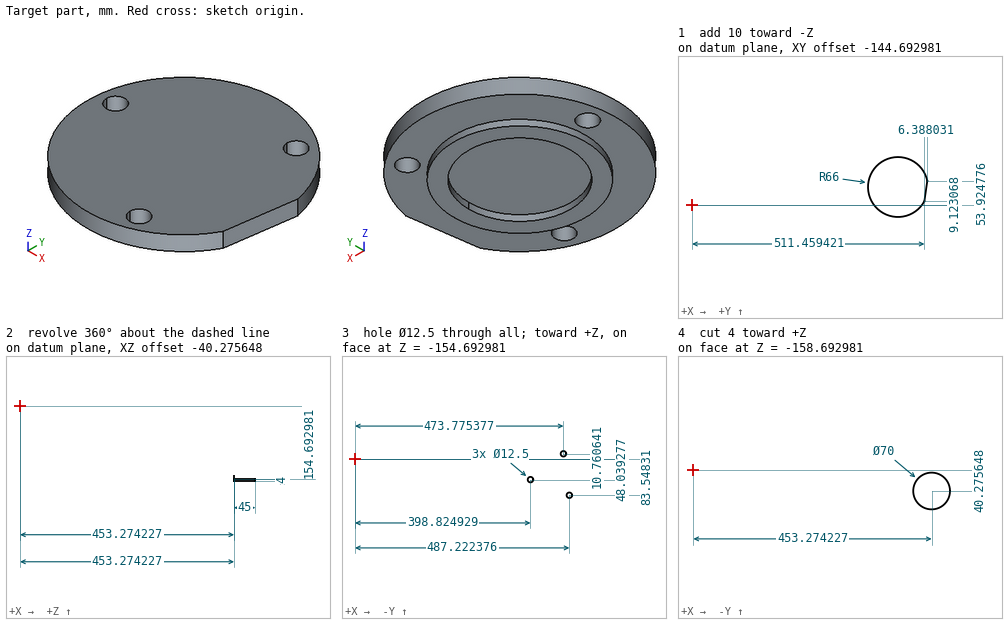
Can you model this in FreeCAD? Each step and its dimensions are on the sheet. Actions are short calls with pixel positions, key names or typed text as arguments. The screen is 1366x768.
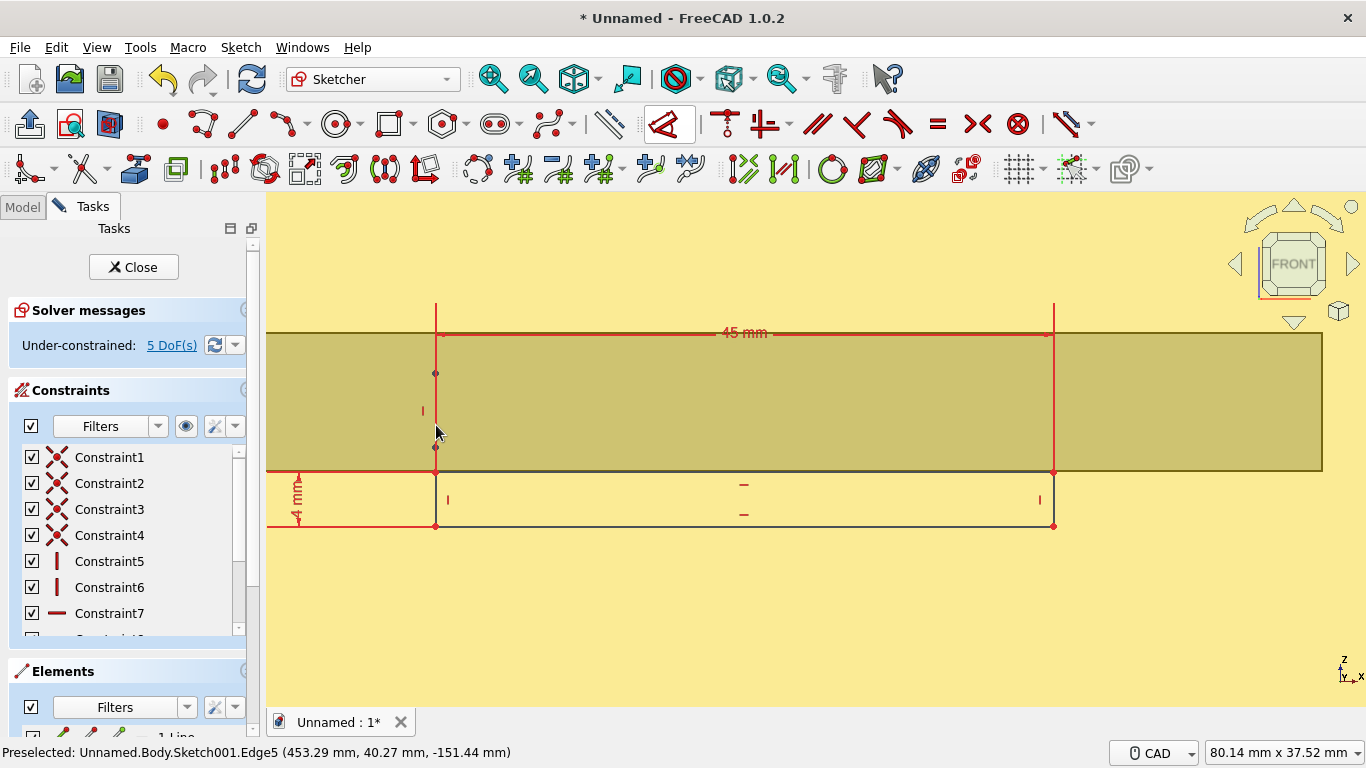
key(g)
key(n)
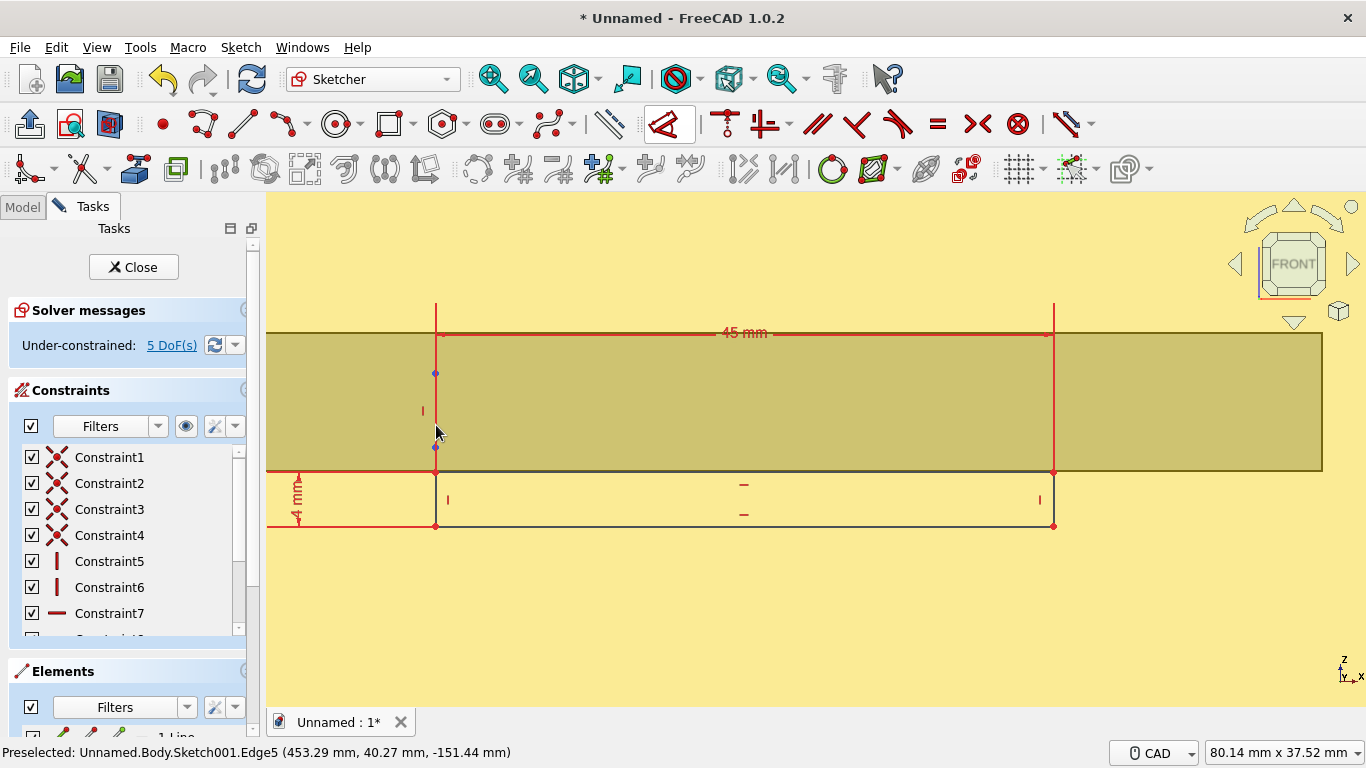
click(436, 472)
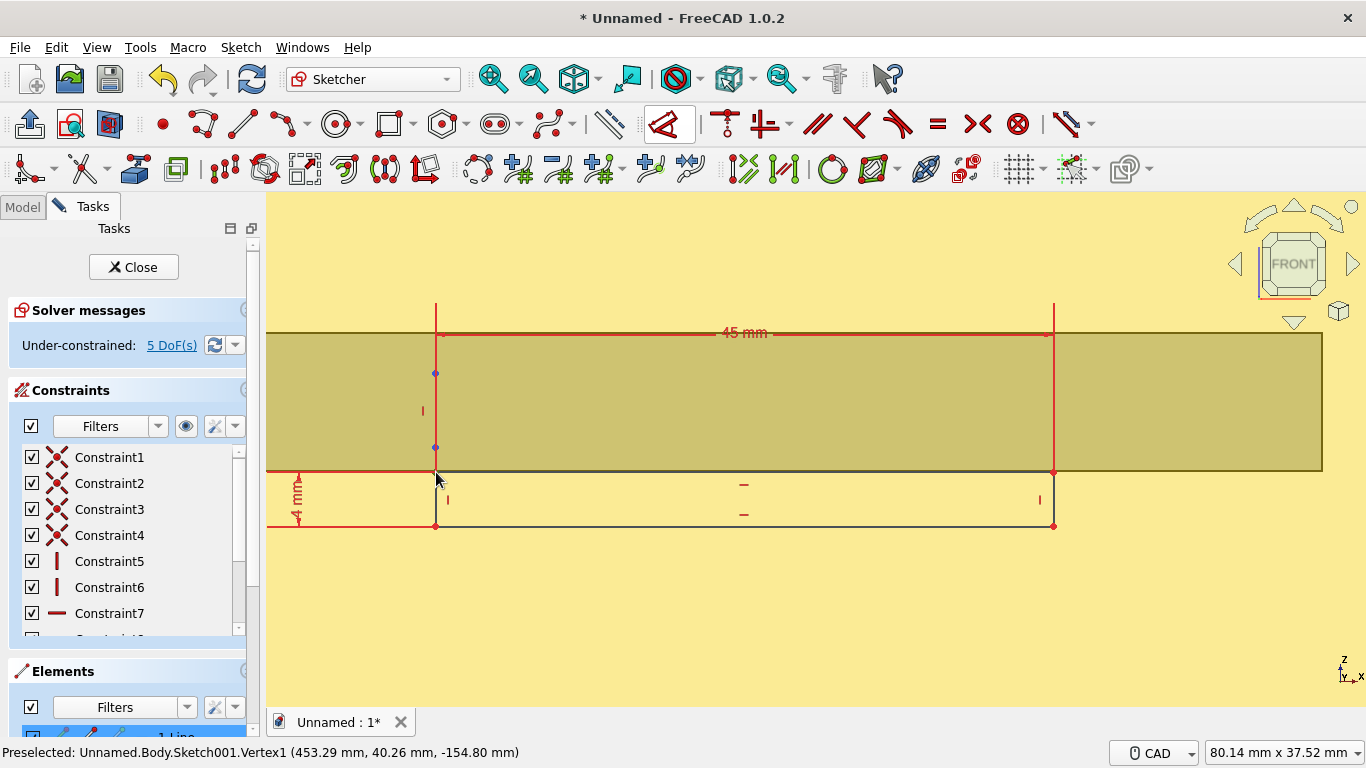
key(l)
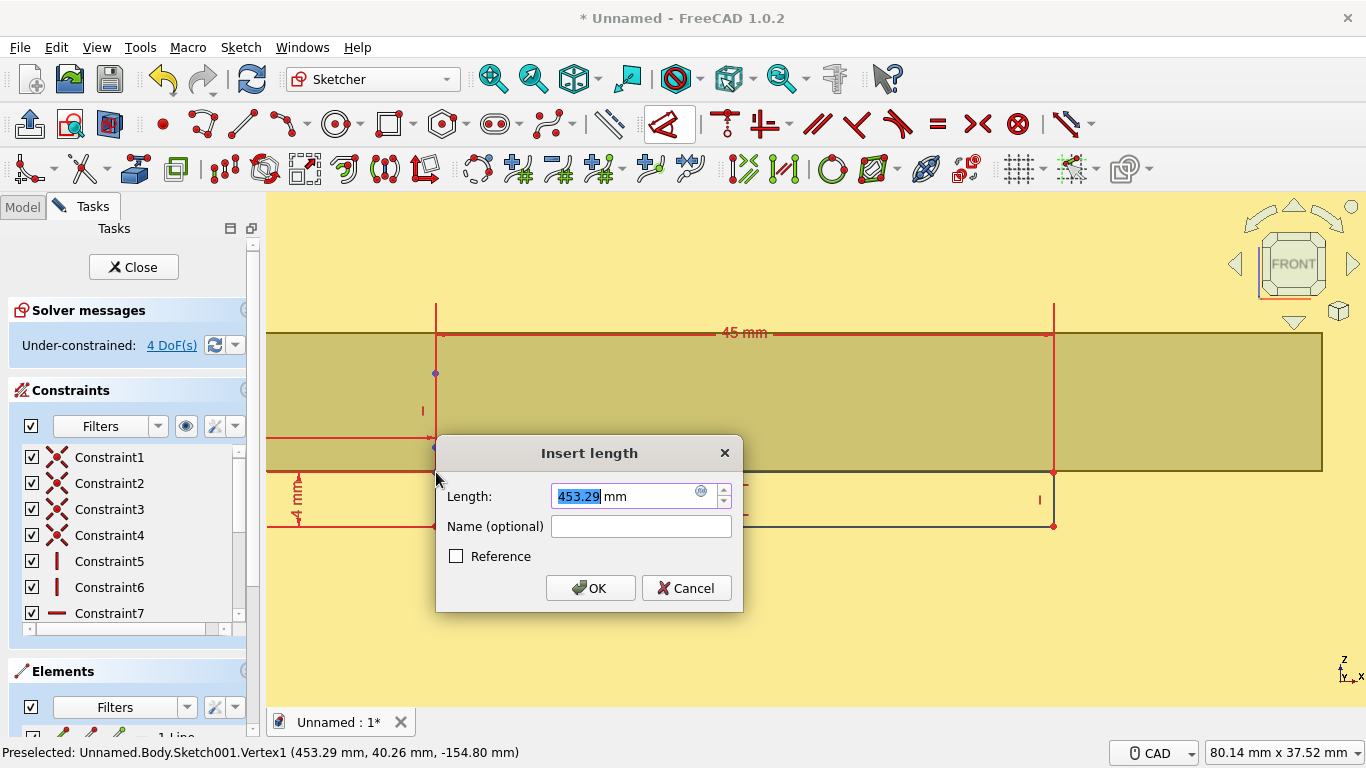
text(453.274227)
key(Return)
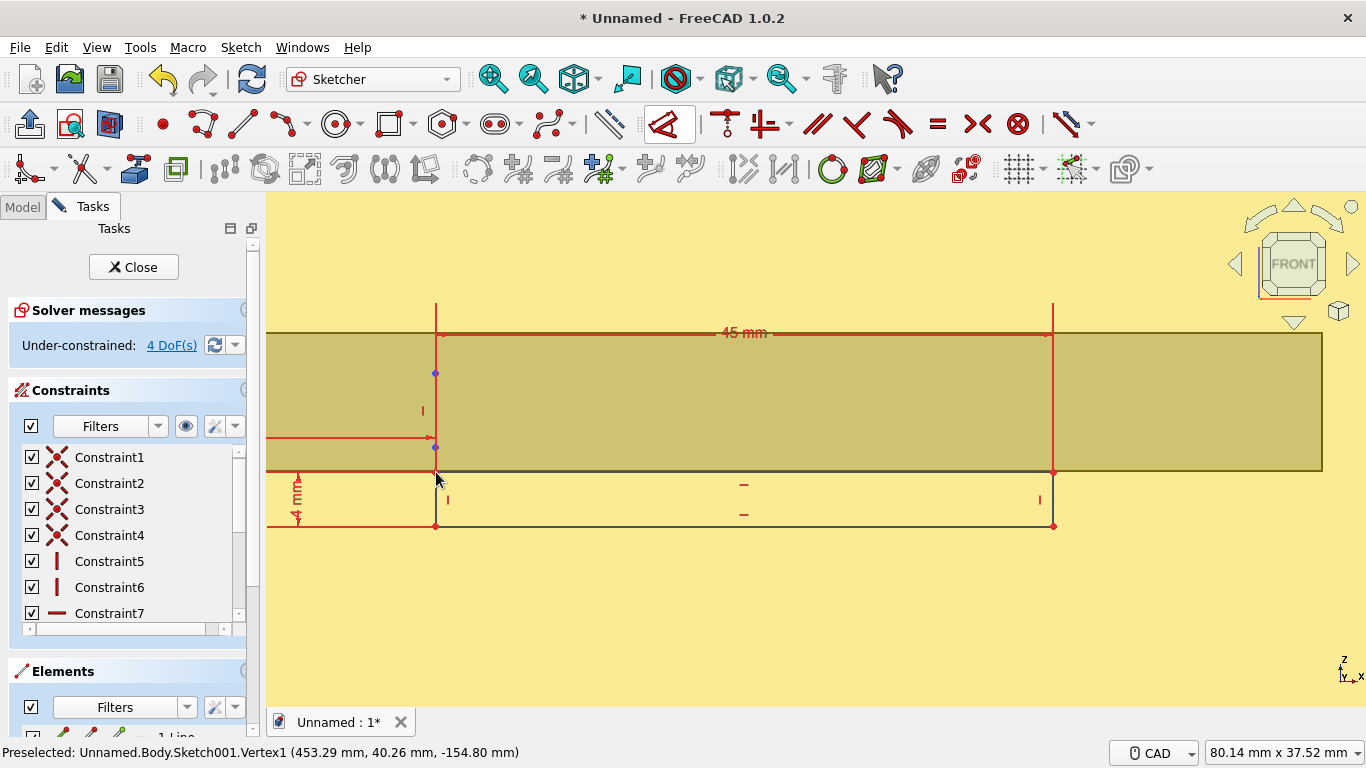
click(436, 472)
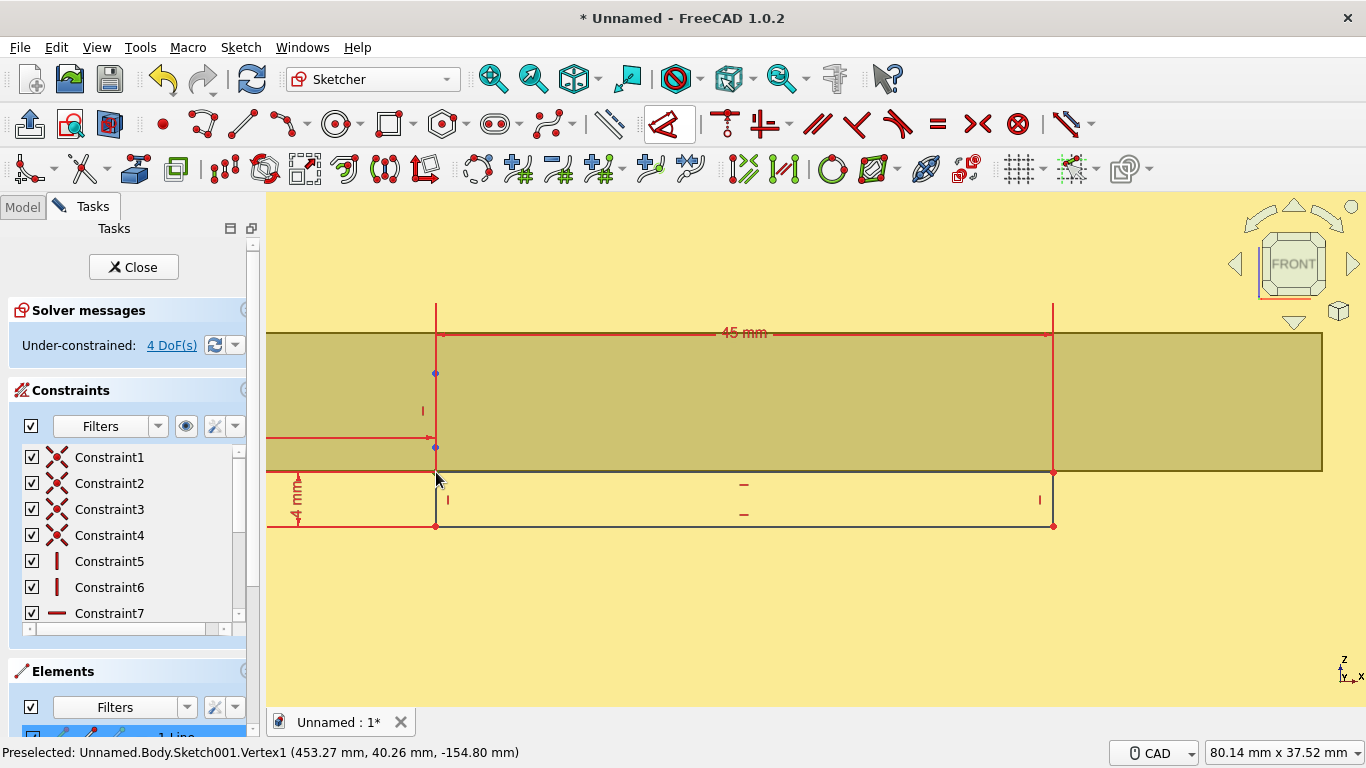
click(690, 124)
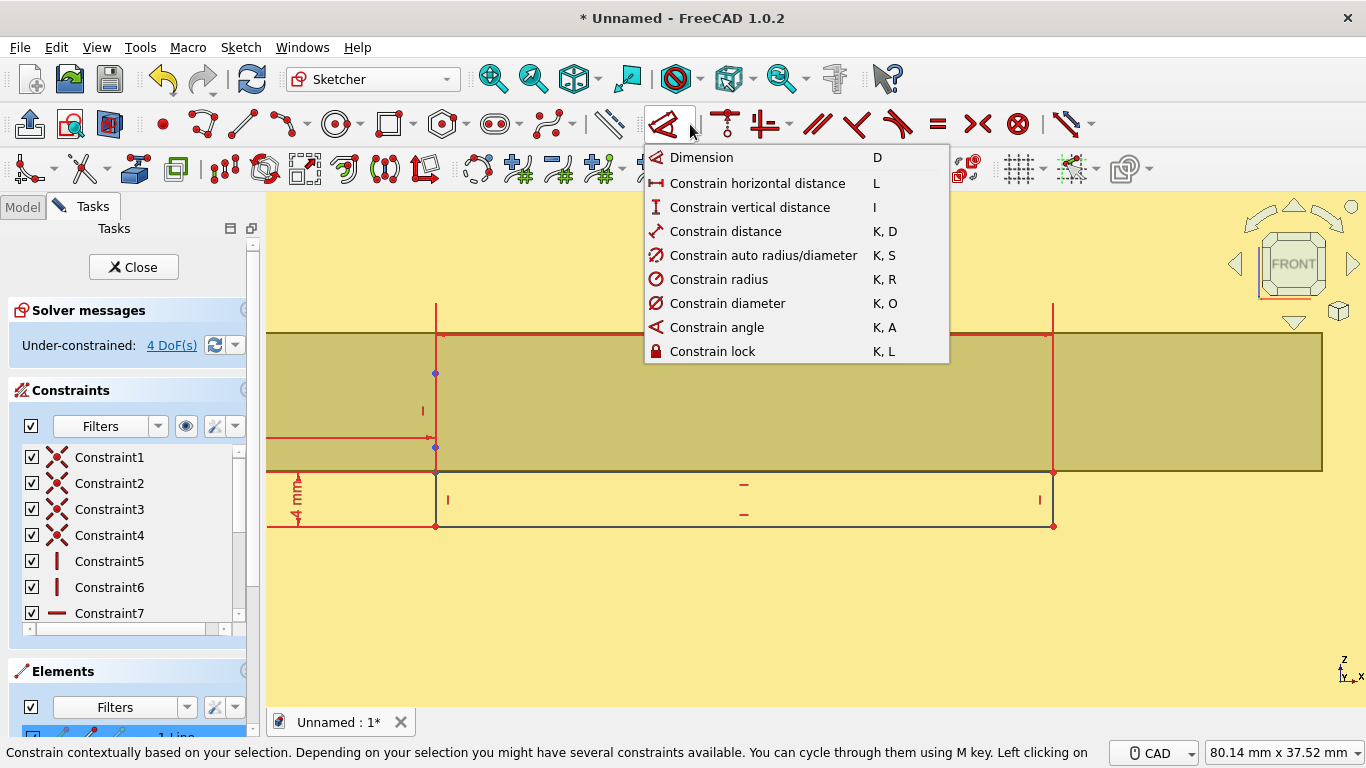
click(797, 207)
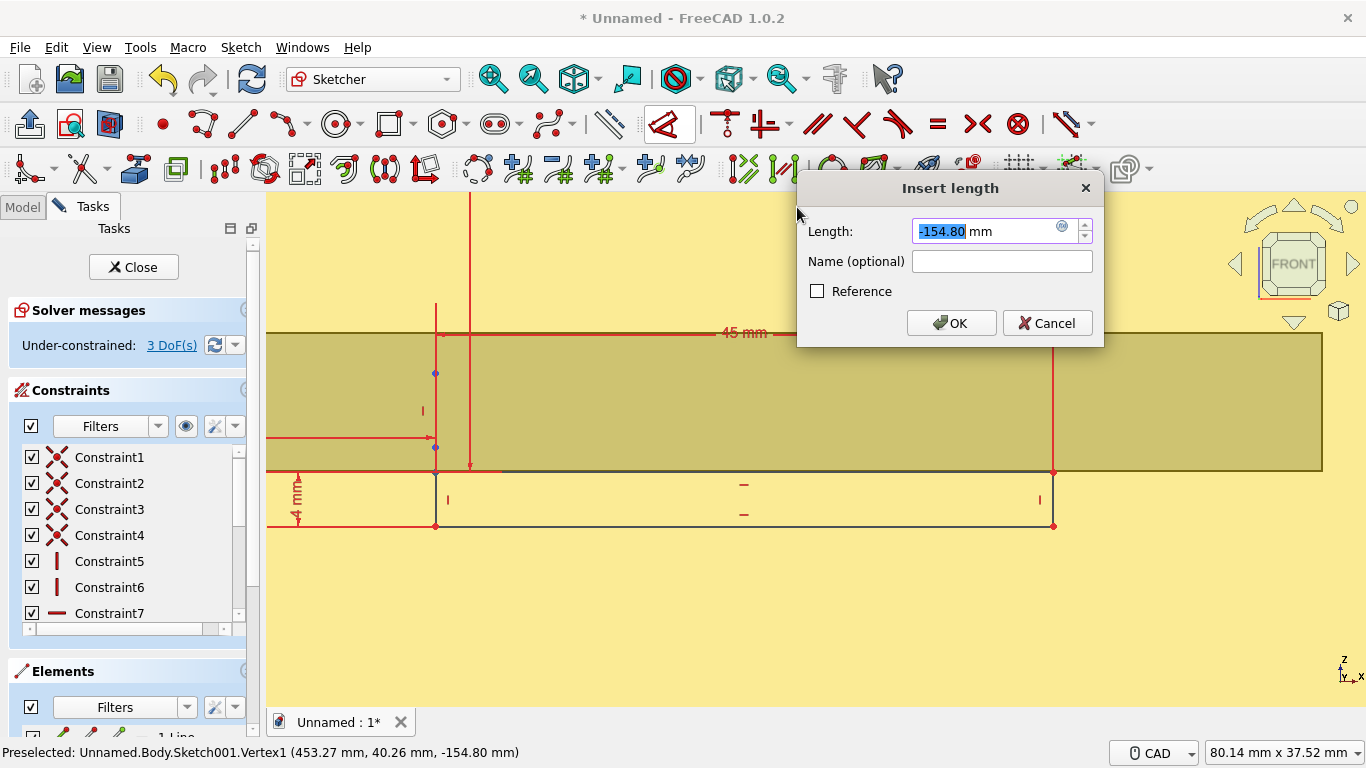
text(-154.692981)
key(Return)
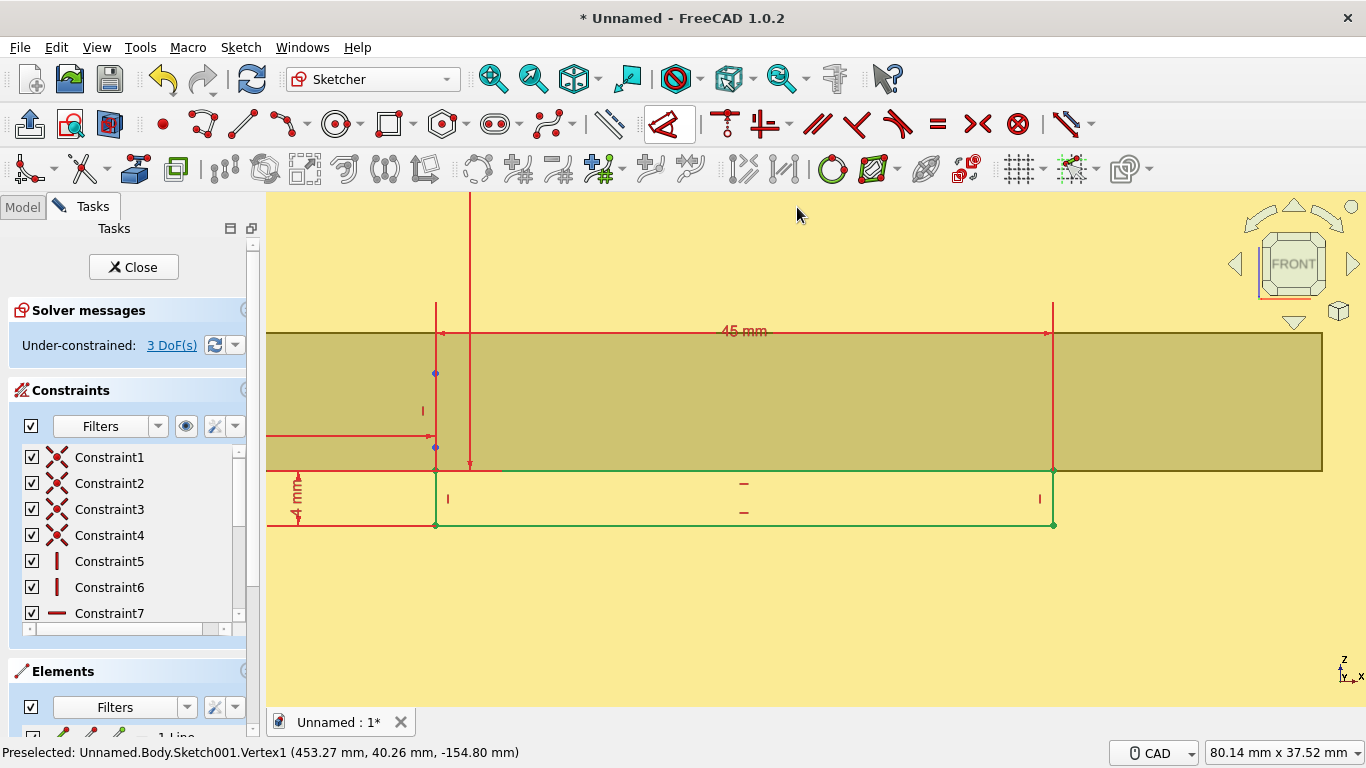
click(436, 447)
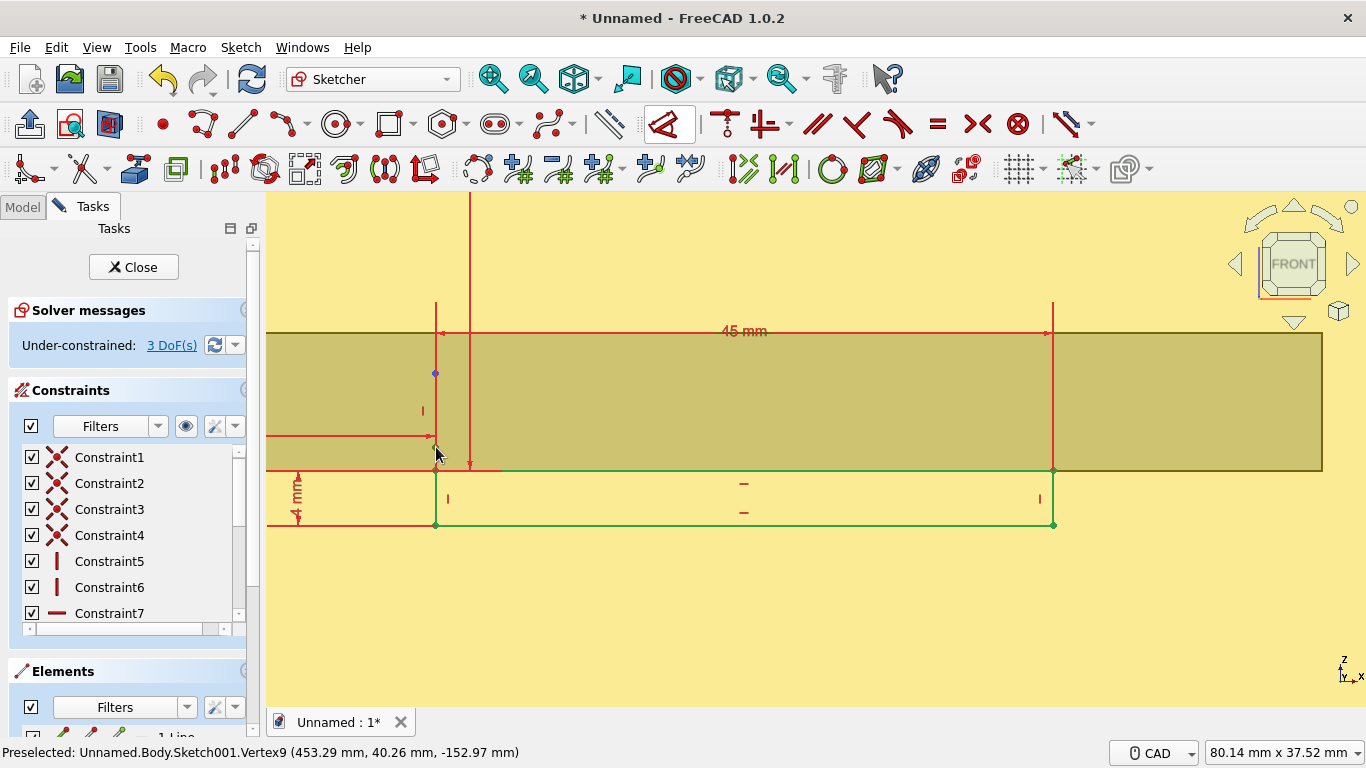
key(l)